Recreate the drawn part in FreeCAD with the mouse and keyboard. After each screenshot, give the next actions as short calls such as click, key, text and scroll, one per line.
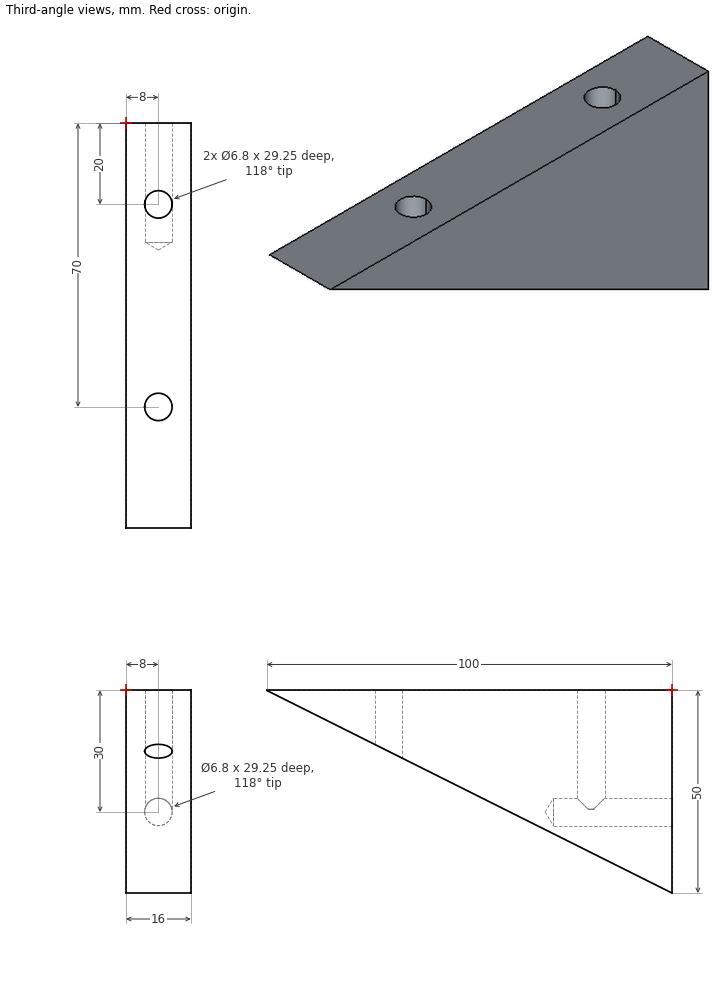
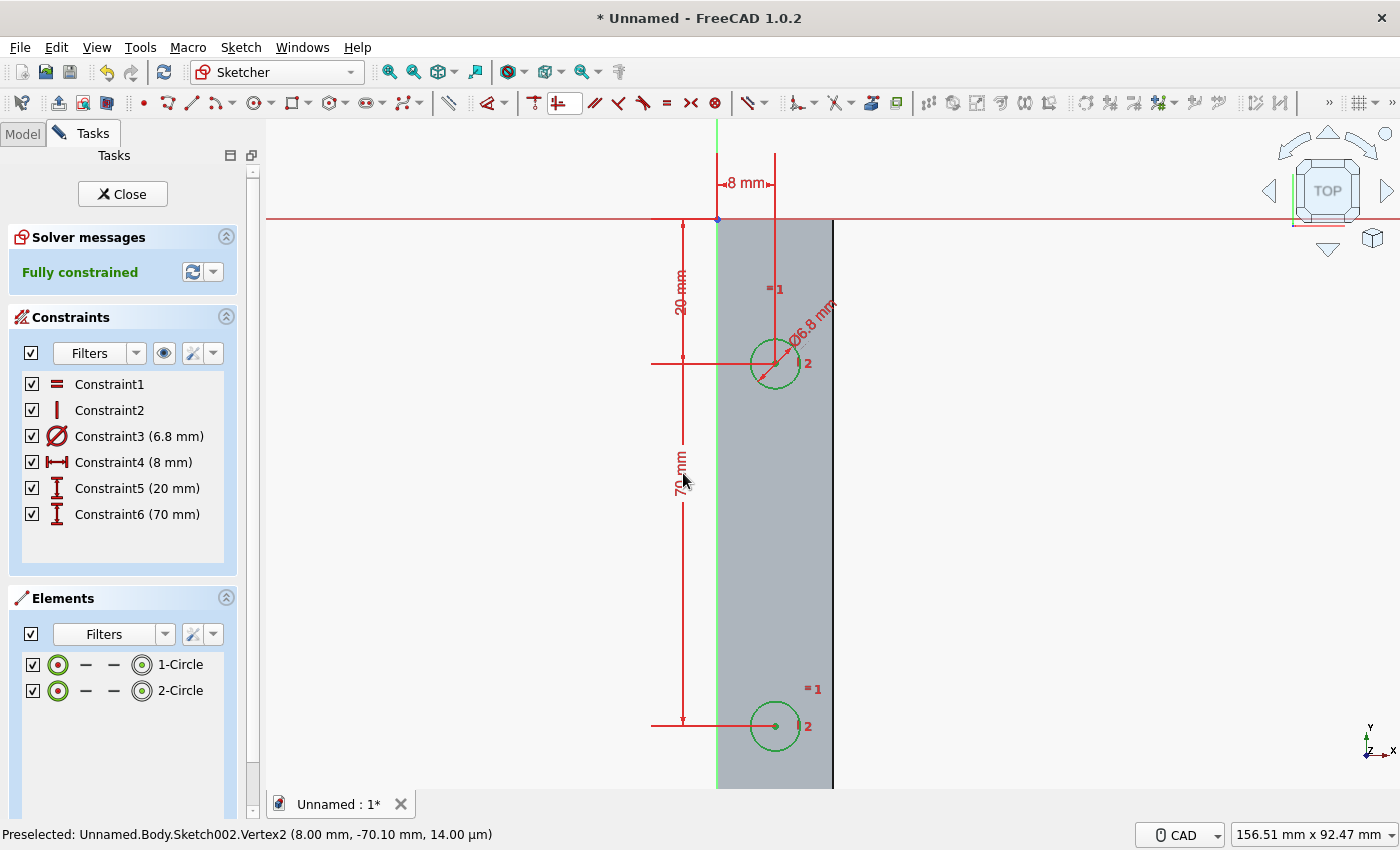
click(123, 194)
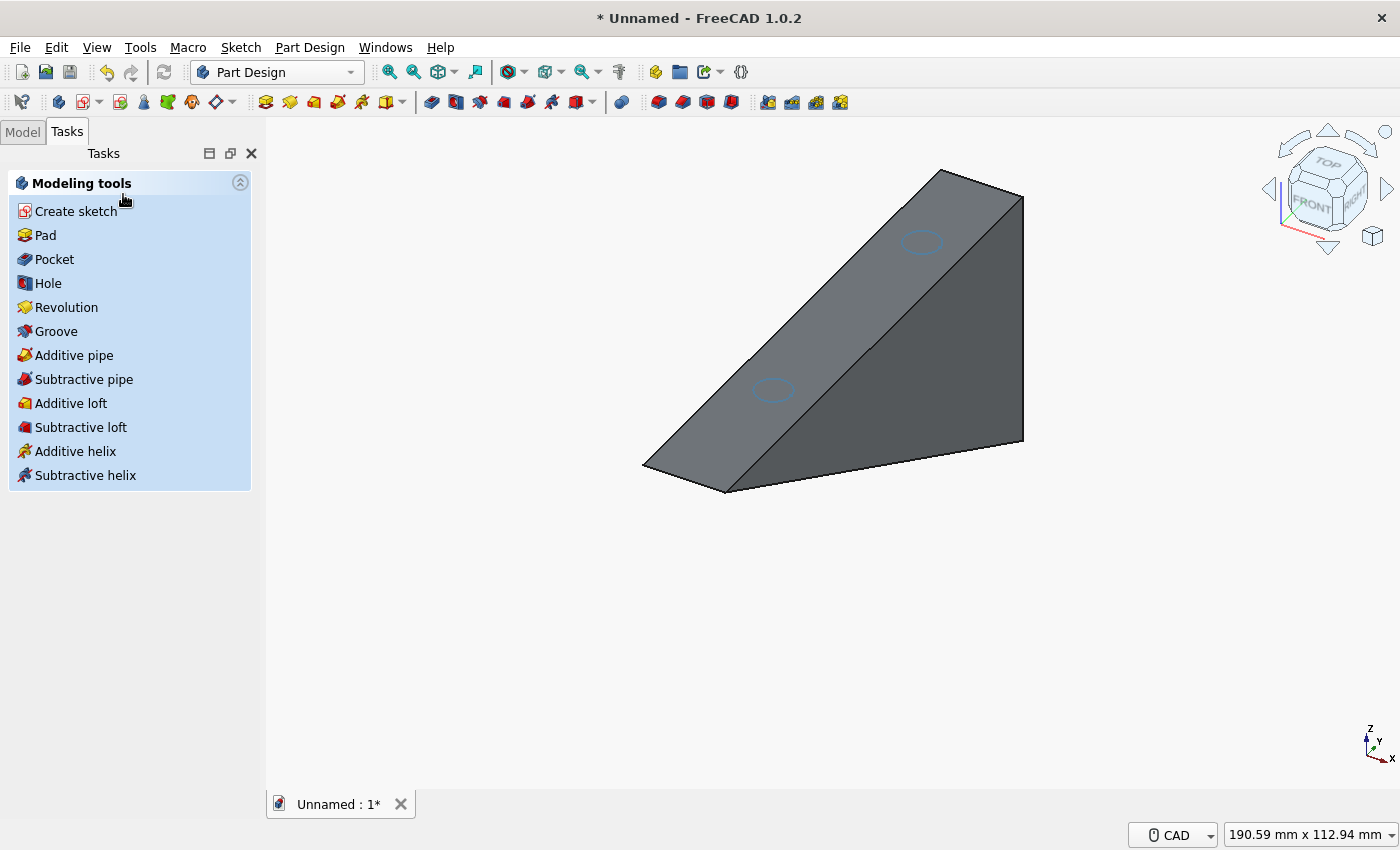
click(456, 102)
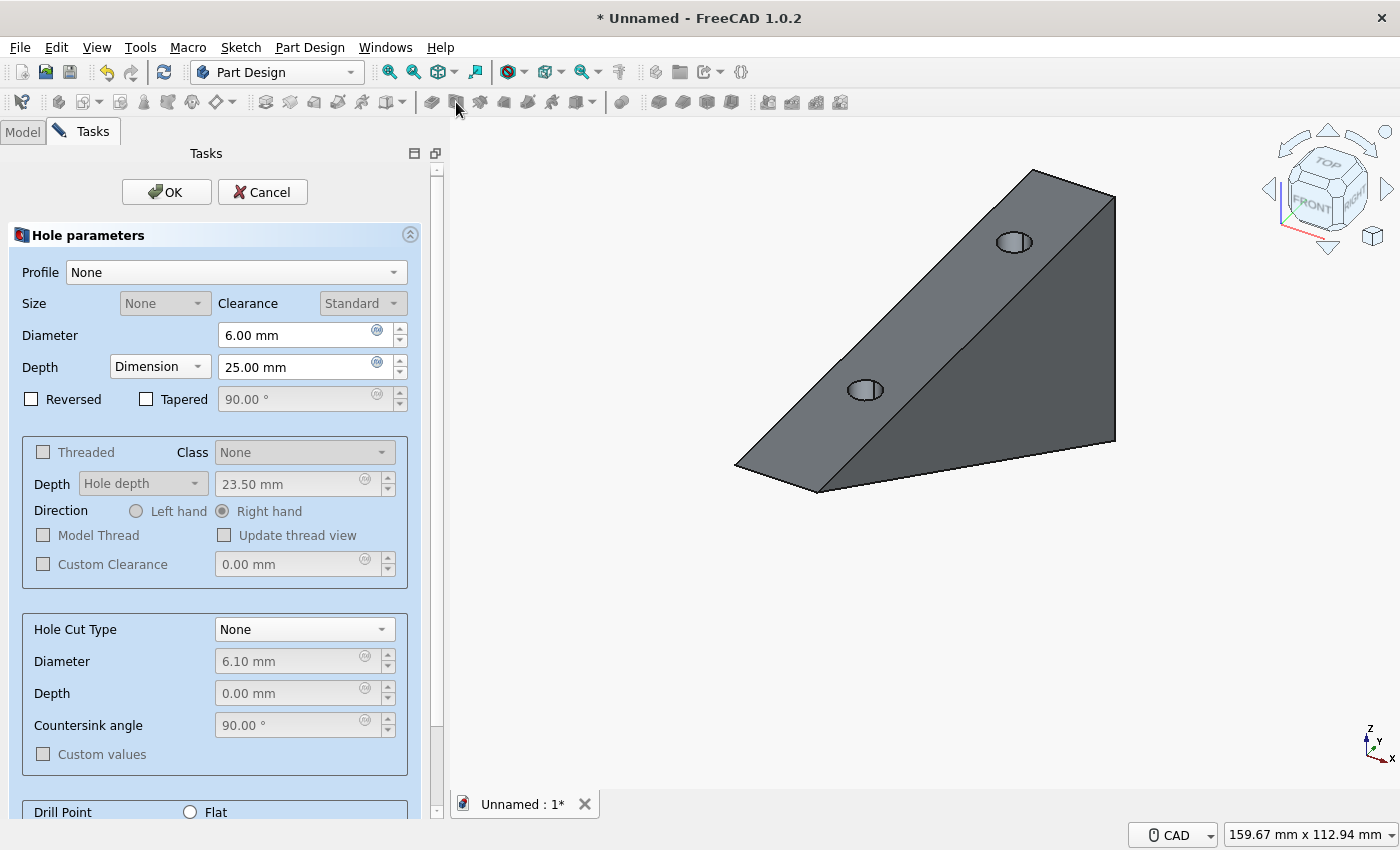
triple_click(305, 335)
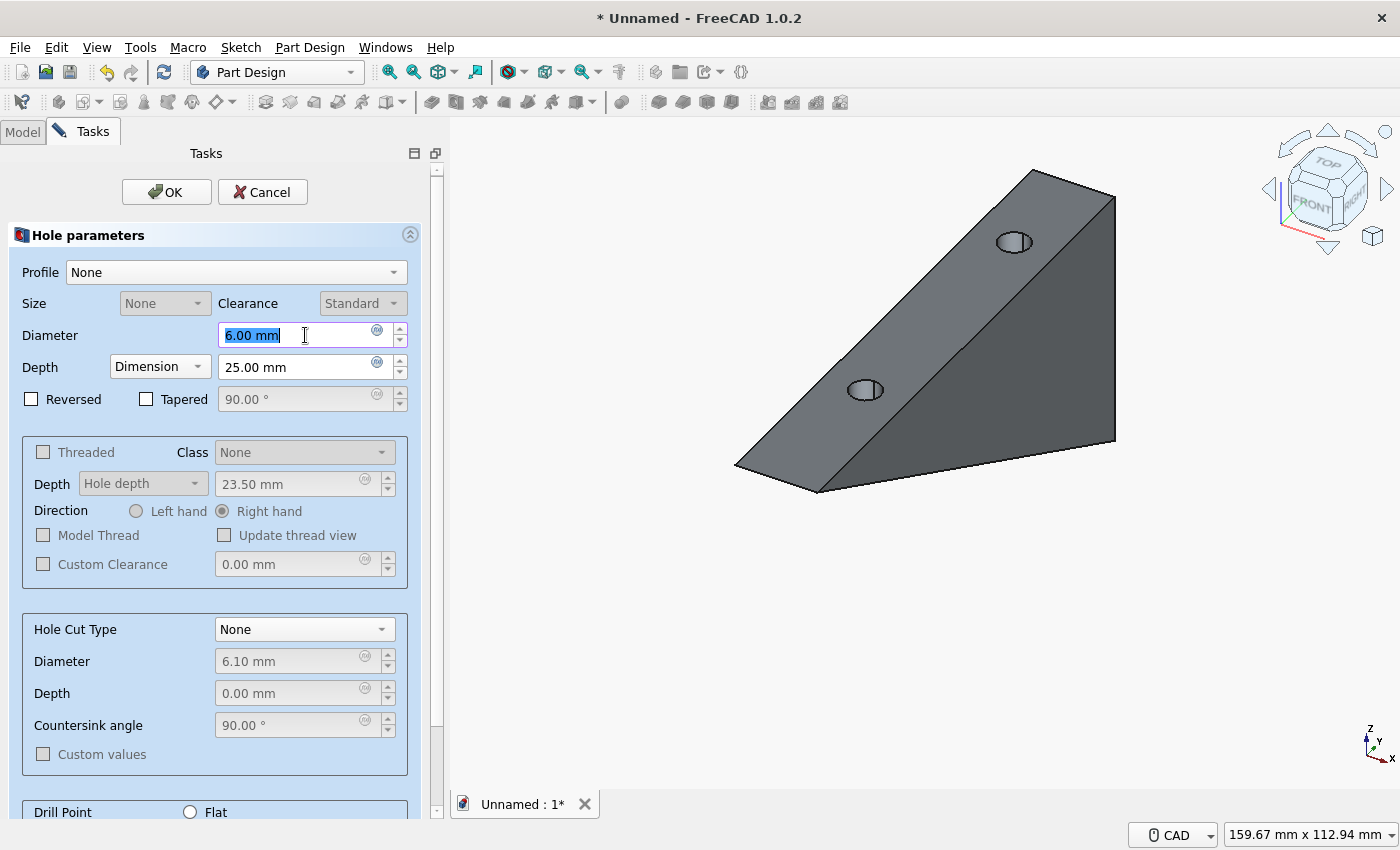
text(6.8)
key(Tab)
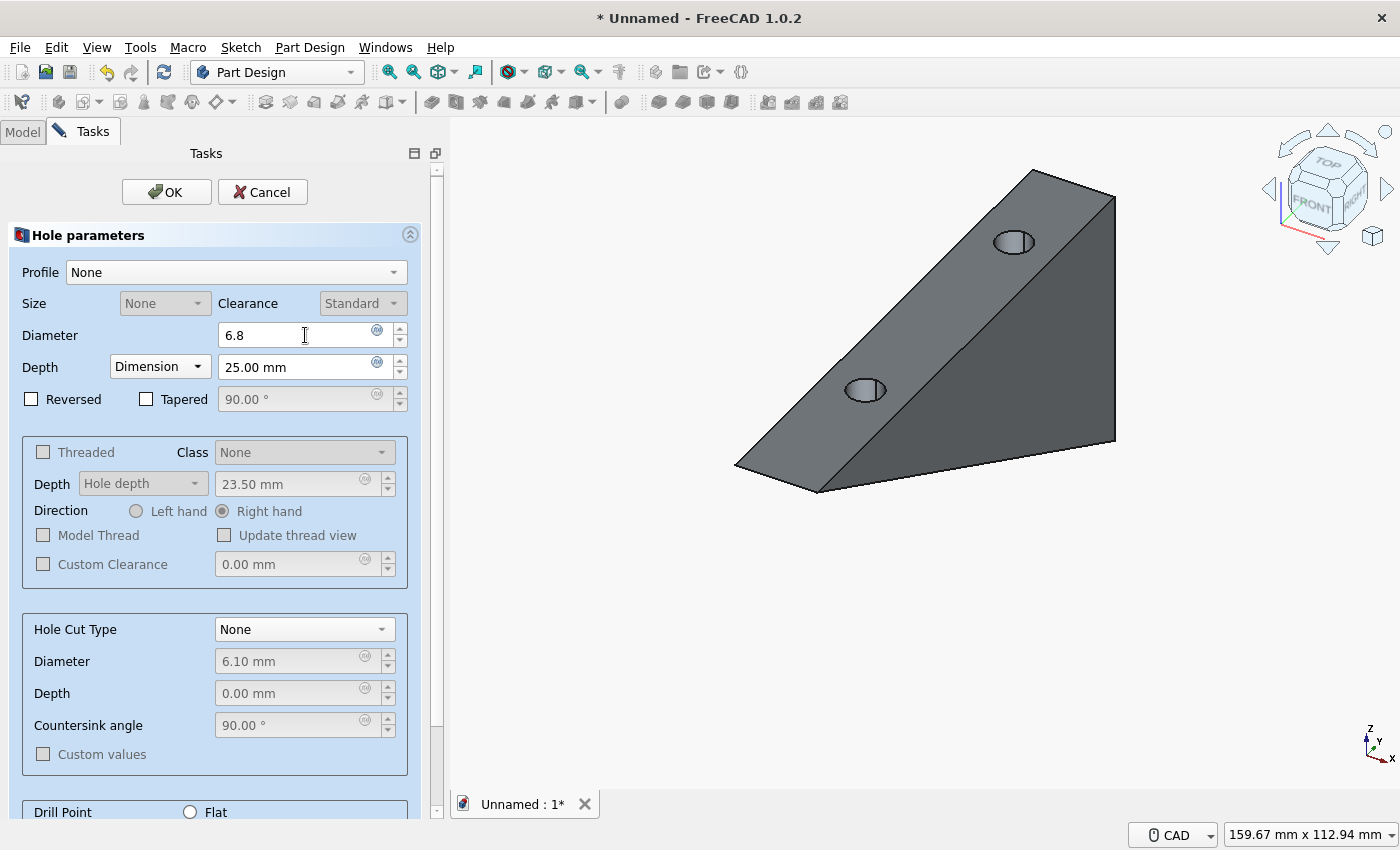
triple_click(305, 367)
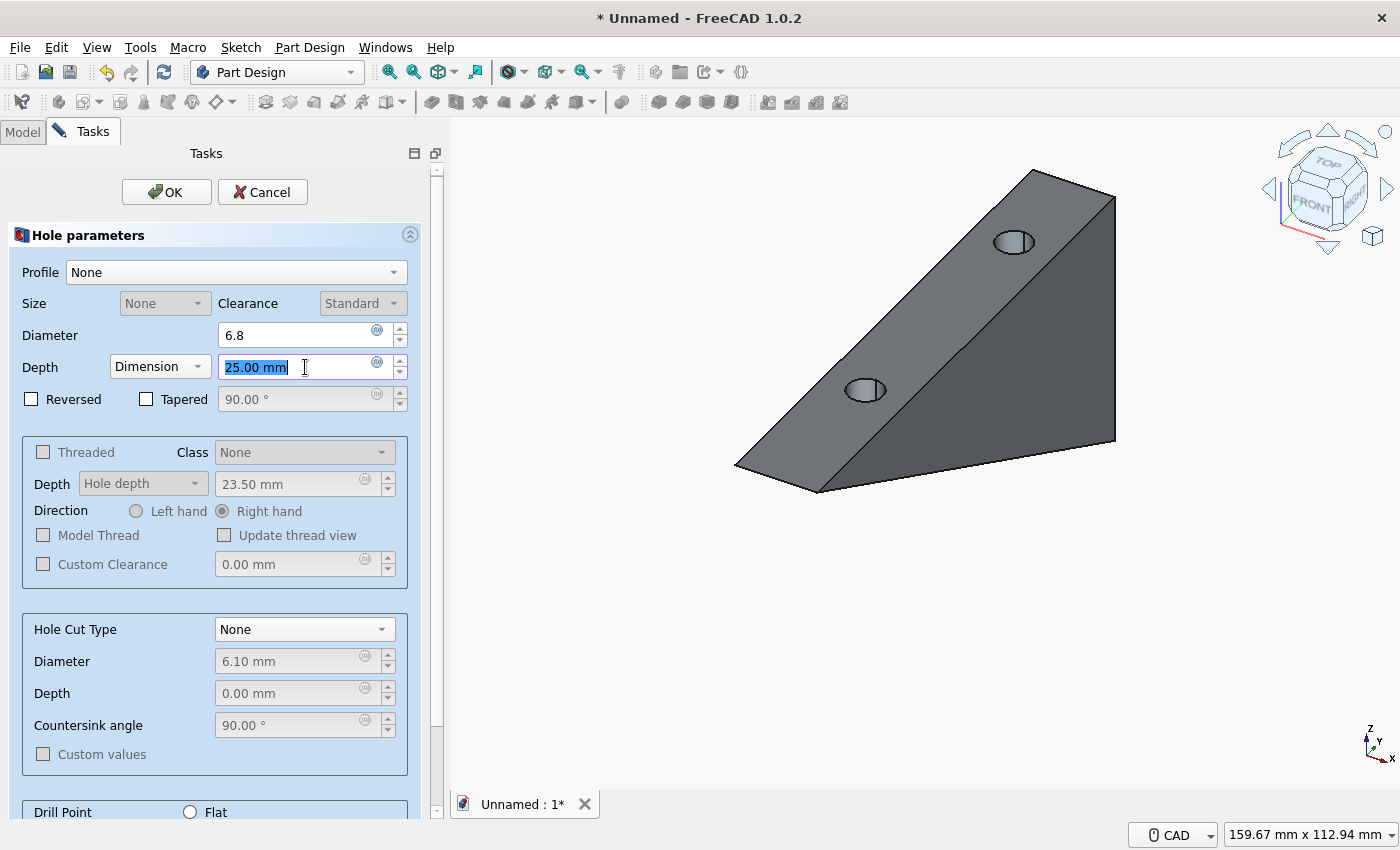
text(29.25)
key(Tab)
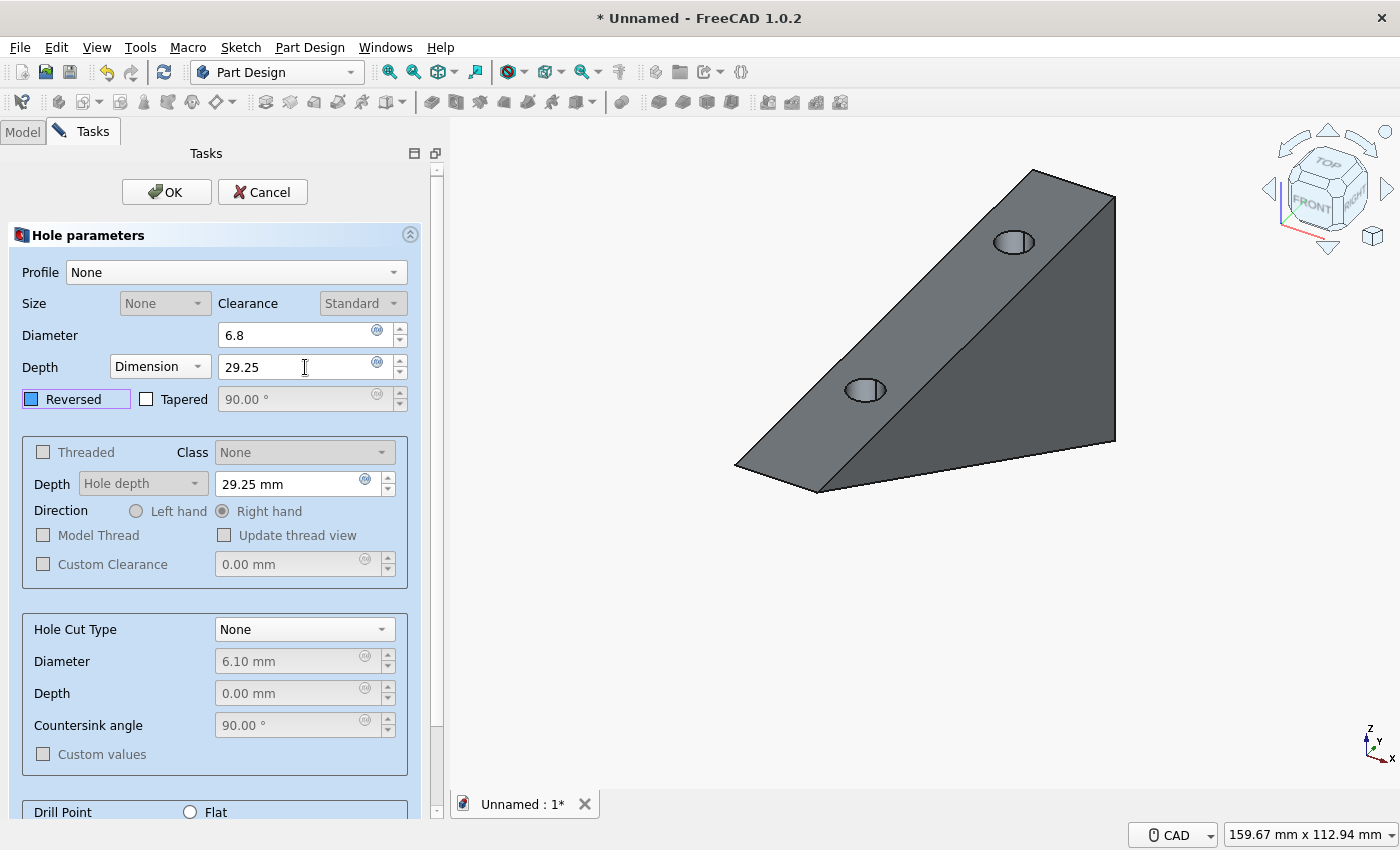
click(167, 192)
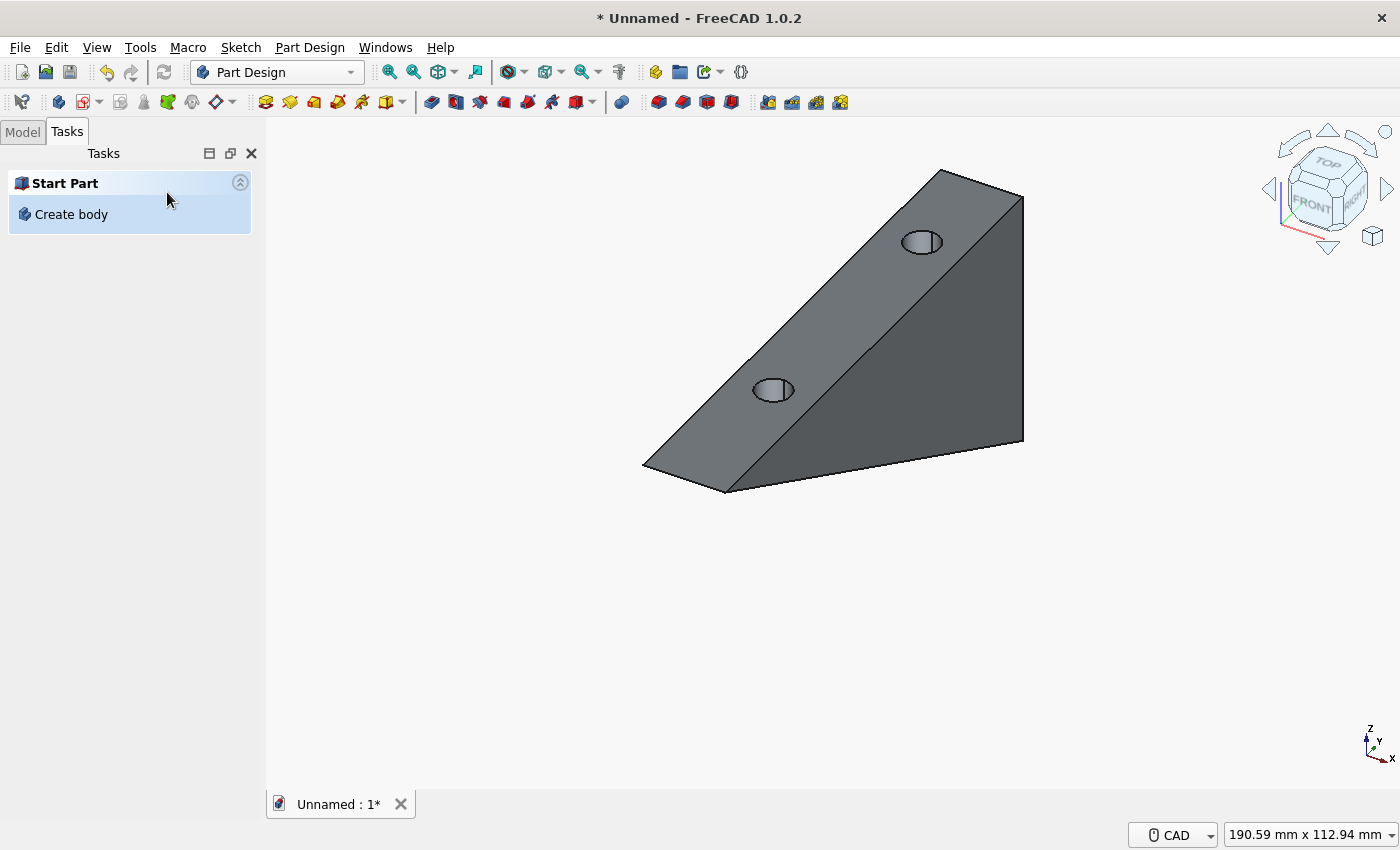
key(0)